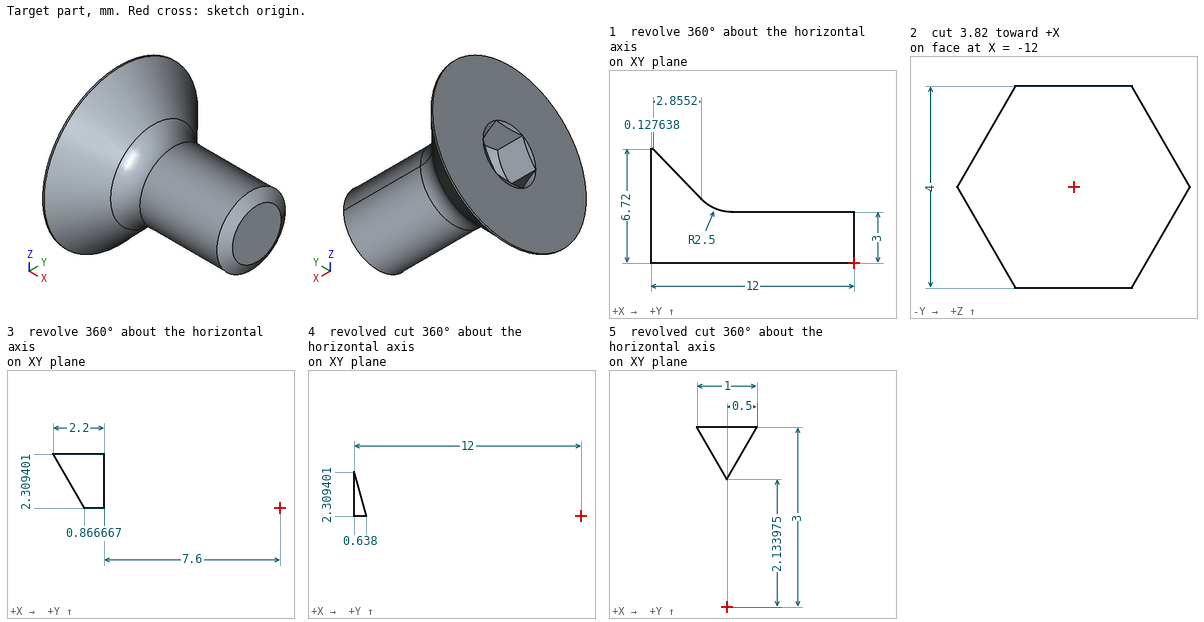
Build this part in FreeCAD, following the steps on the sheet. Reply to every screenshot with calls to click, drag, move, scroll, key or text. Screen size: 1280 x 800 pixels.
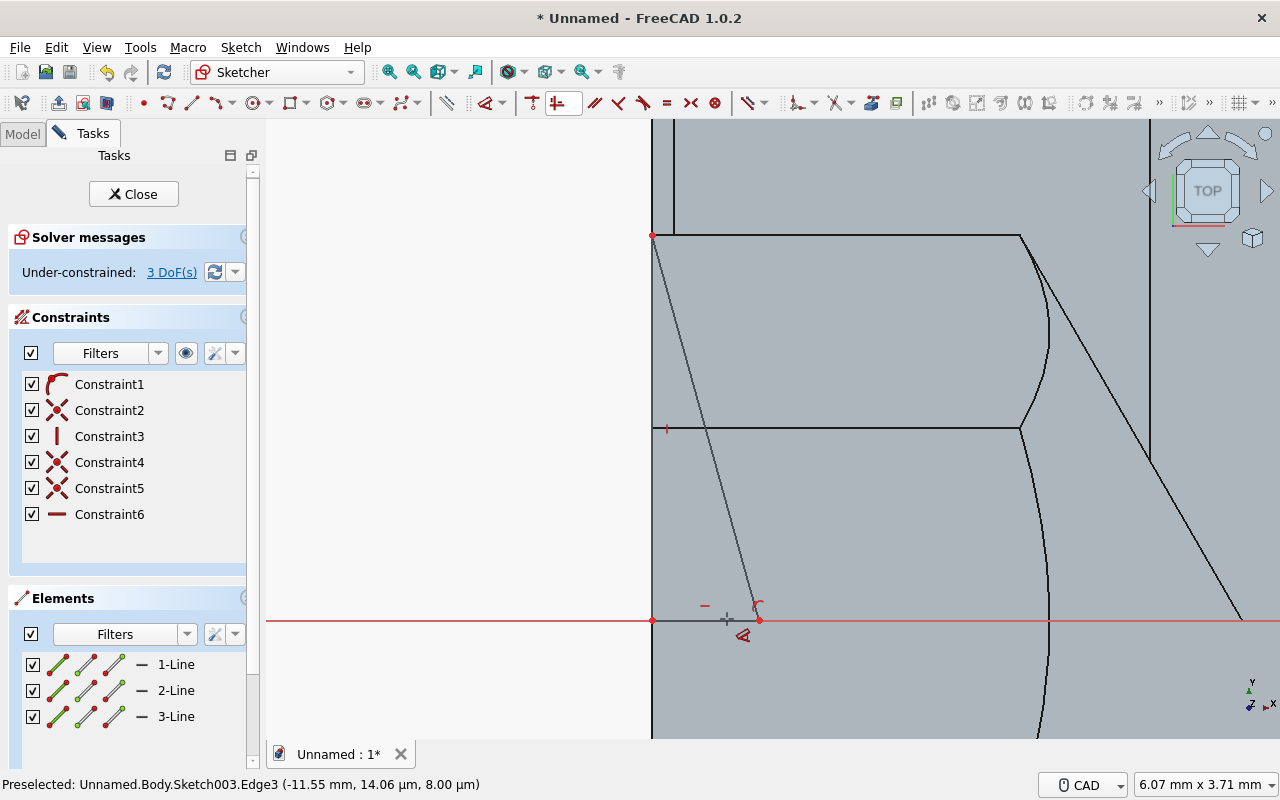
click(652, 236)
click(883, 655)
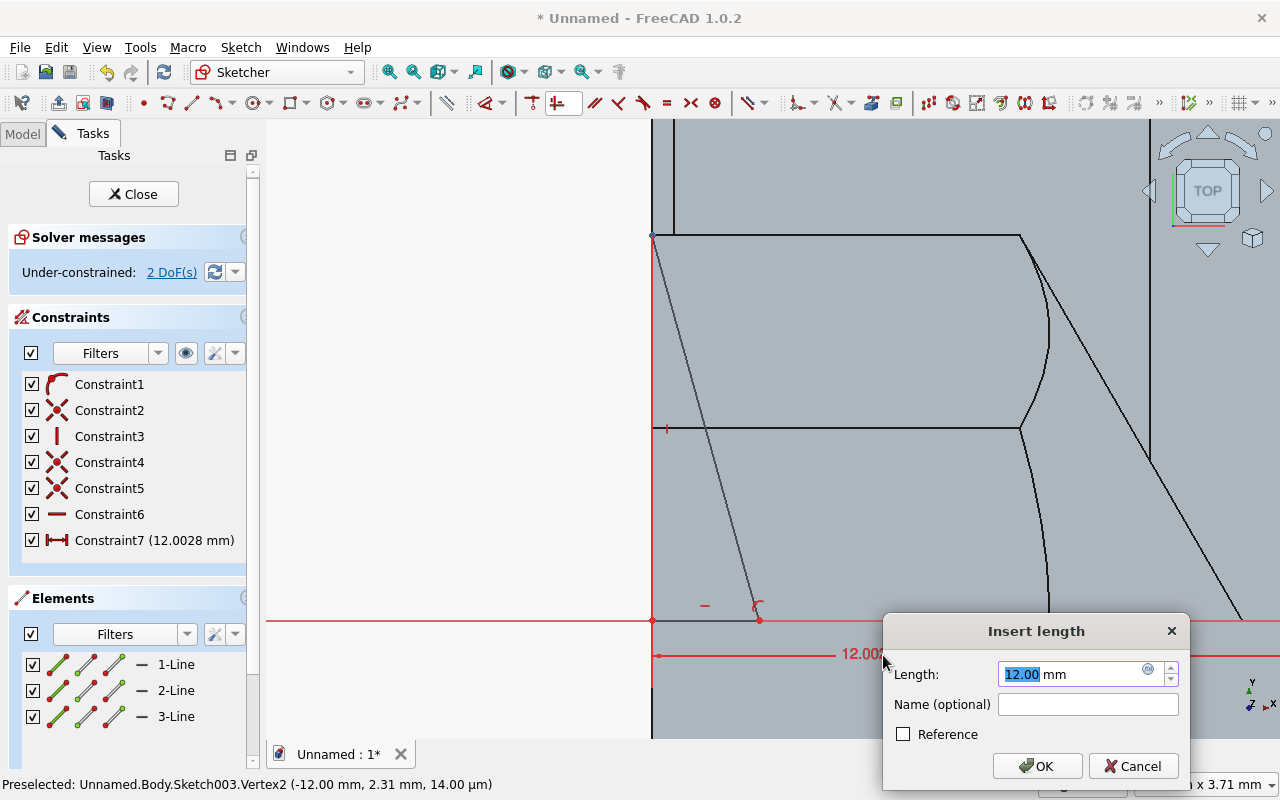
text(12)
key(Return)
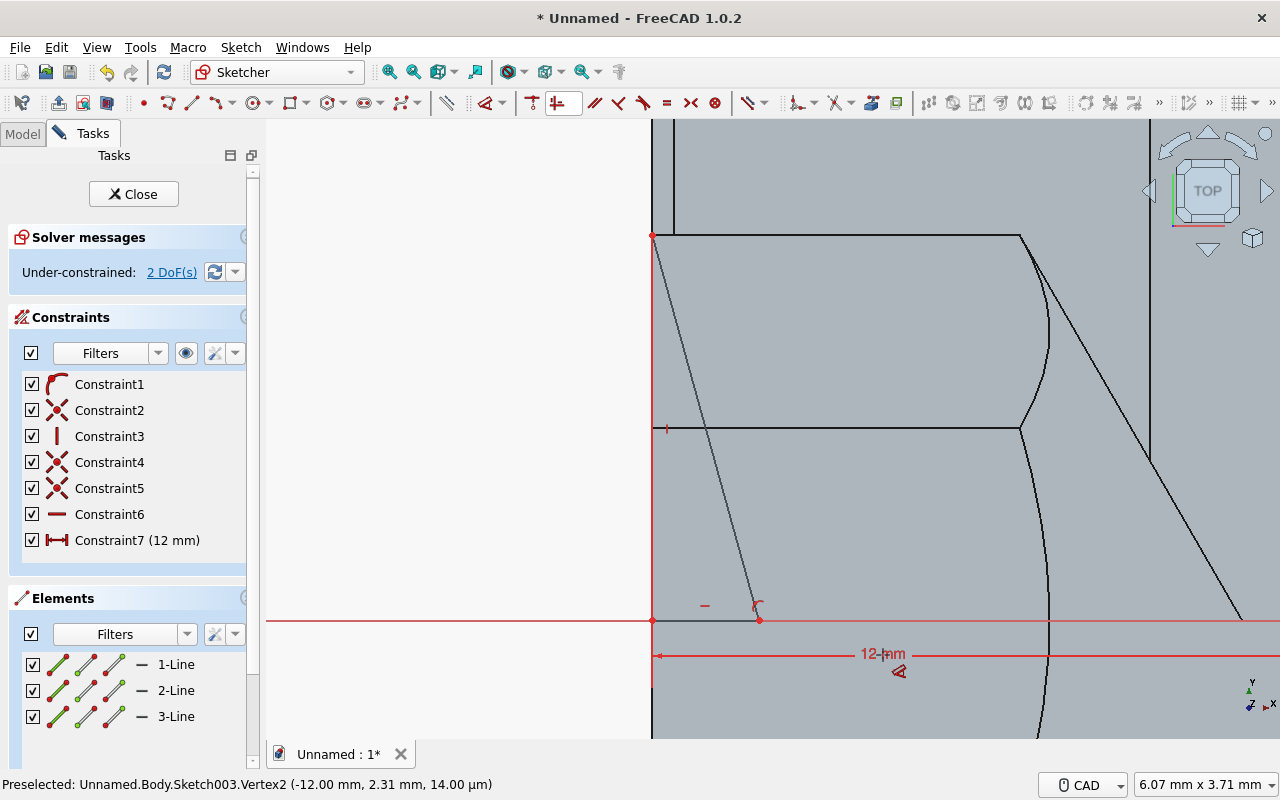
click(684, 621)
click(706, 655)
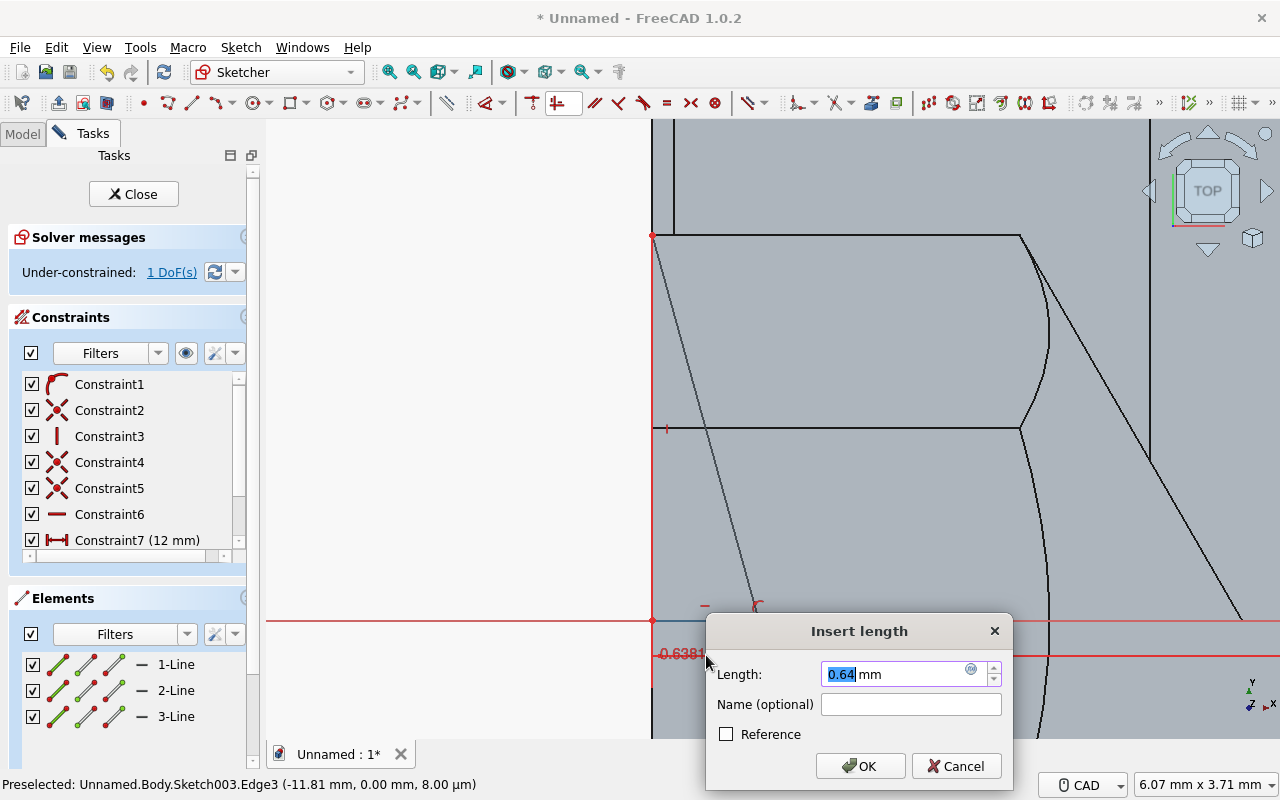
text(0.638)
key(Return)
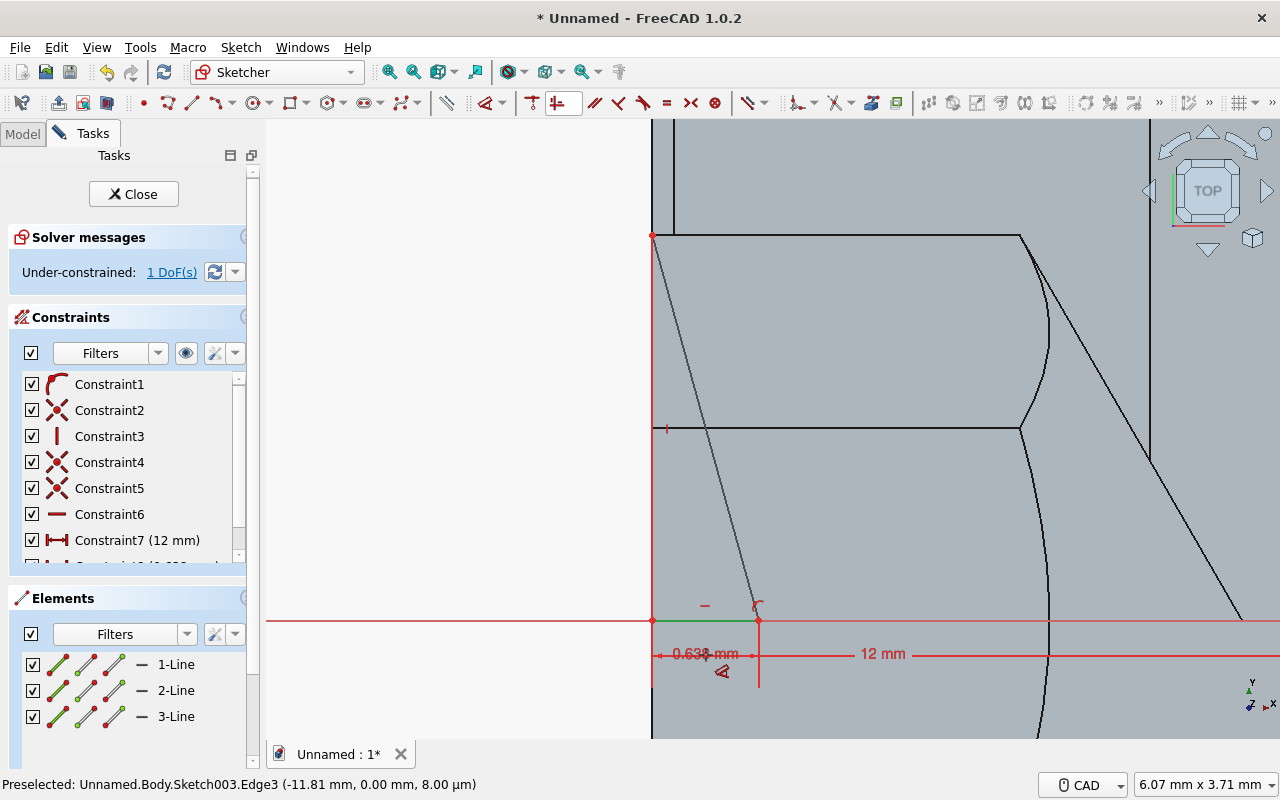
click(652, 351)
click(618, 428)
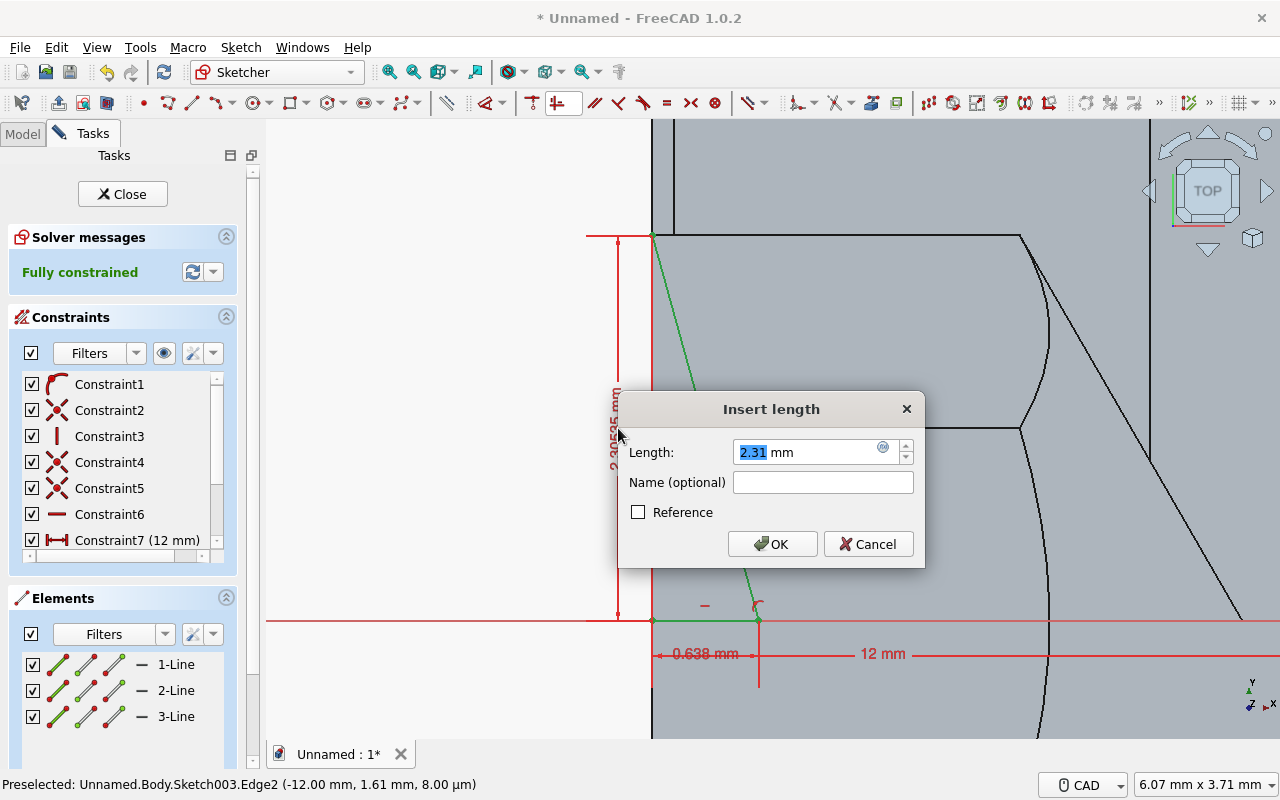
text(2.309401)
key(Return)
key(Escape)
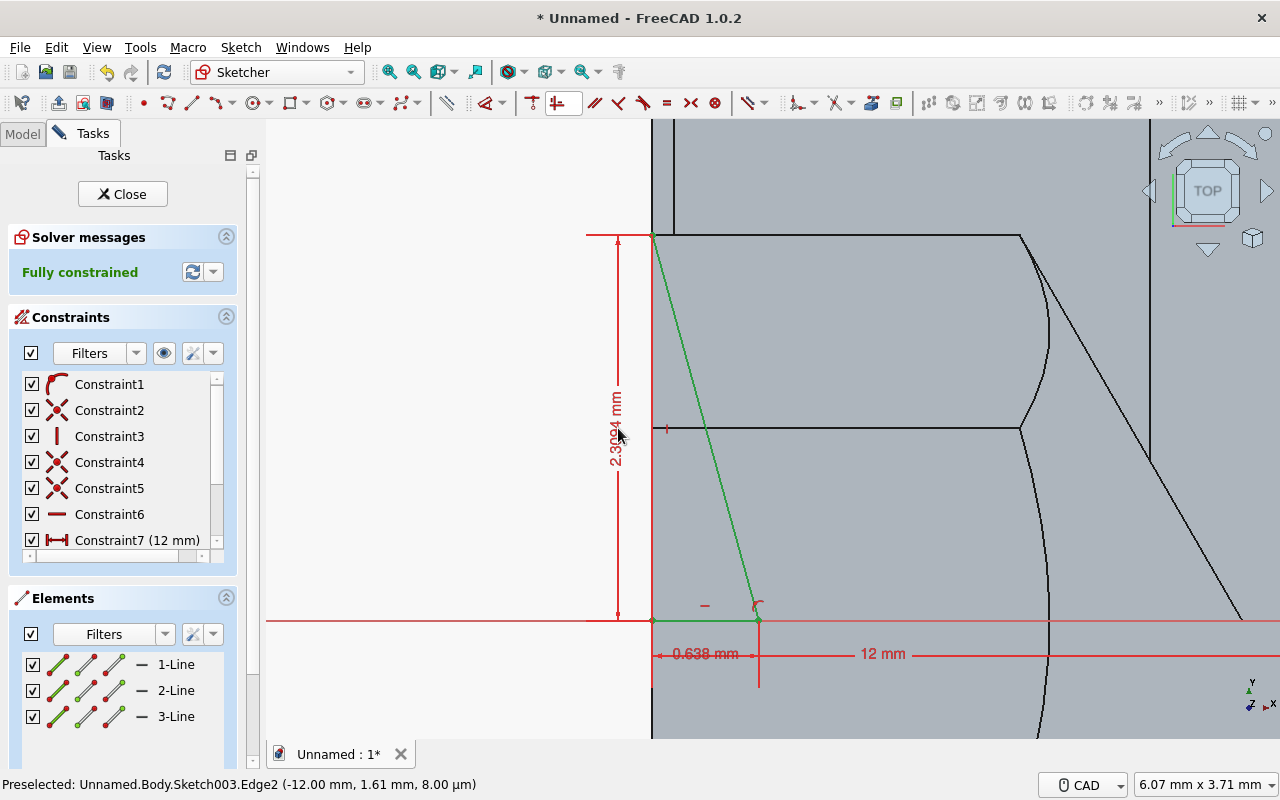
click(123, 194)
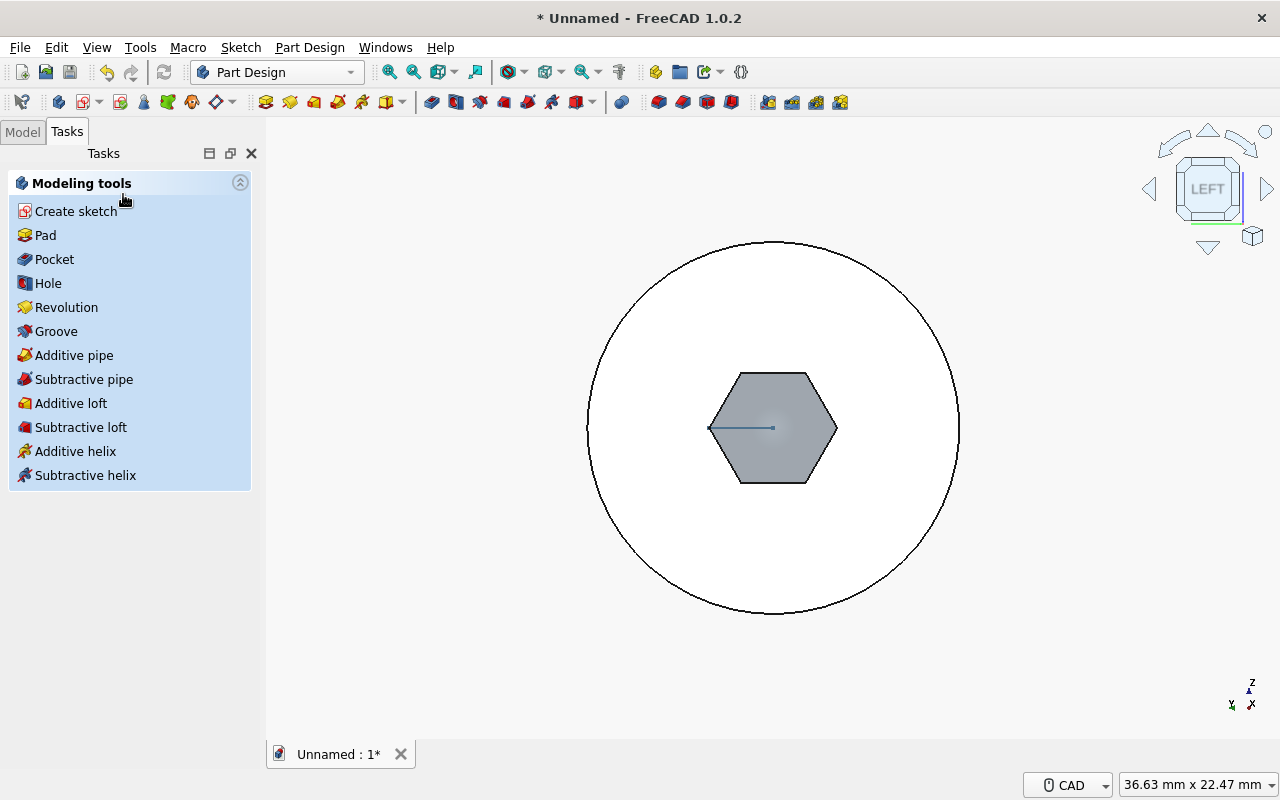
click(480, 102)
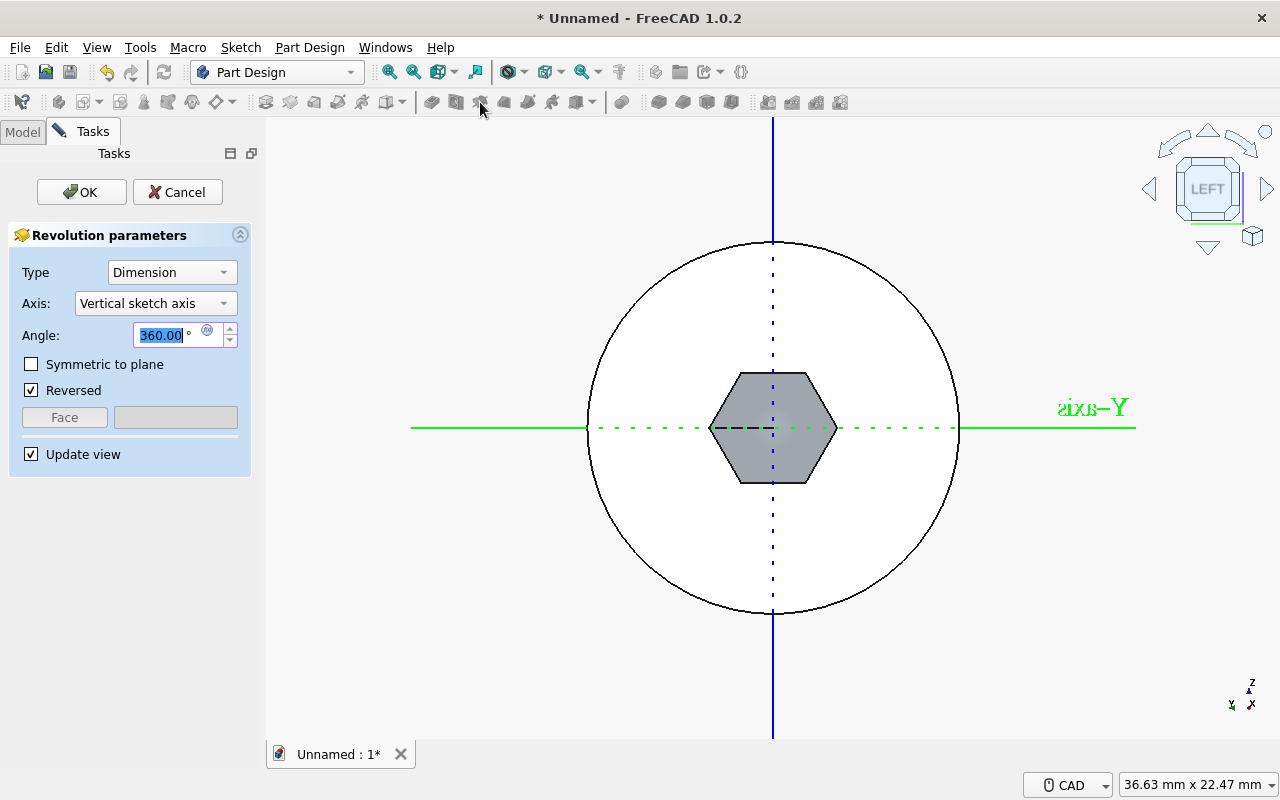
click(156, 304)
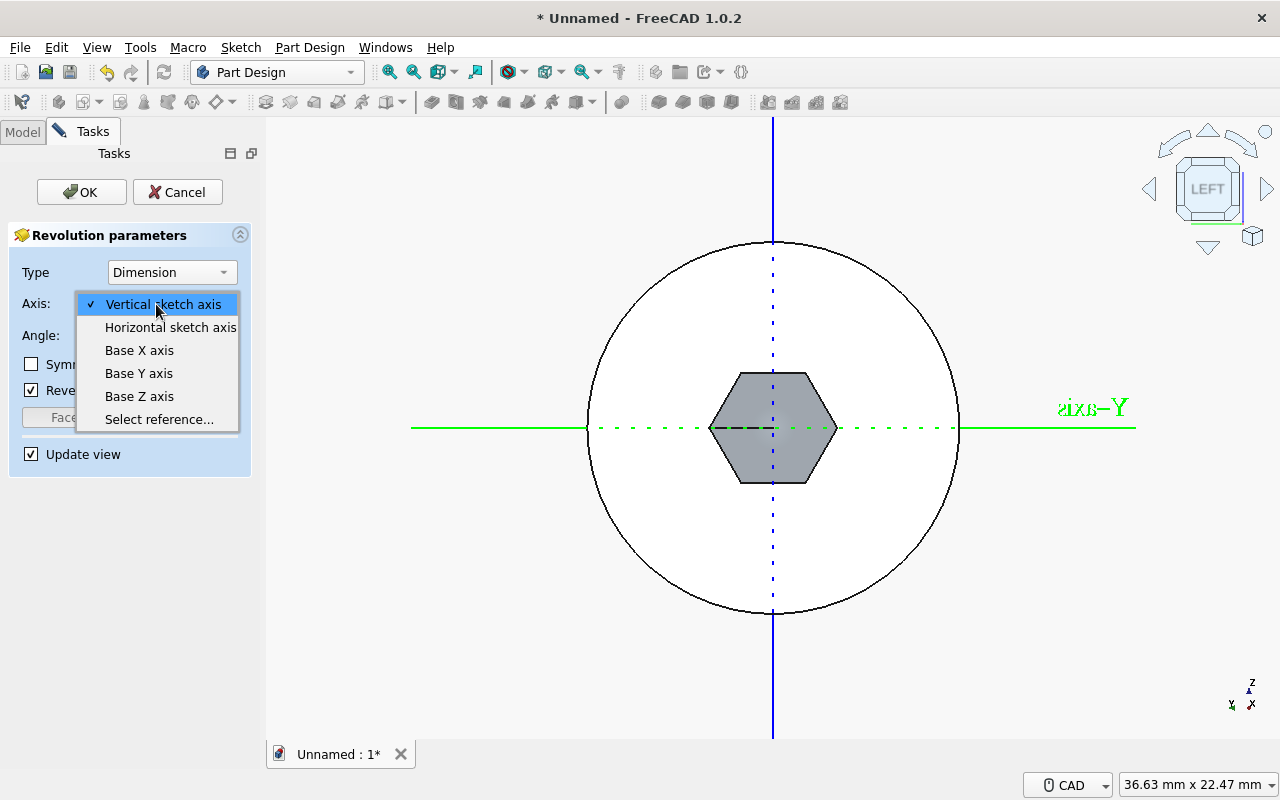
click(156, 328)